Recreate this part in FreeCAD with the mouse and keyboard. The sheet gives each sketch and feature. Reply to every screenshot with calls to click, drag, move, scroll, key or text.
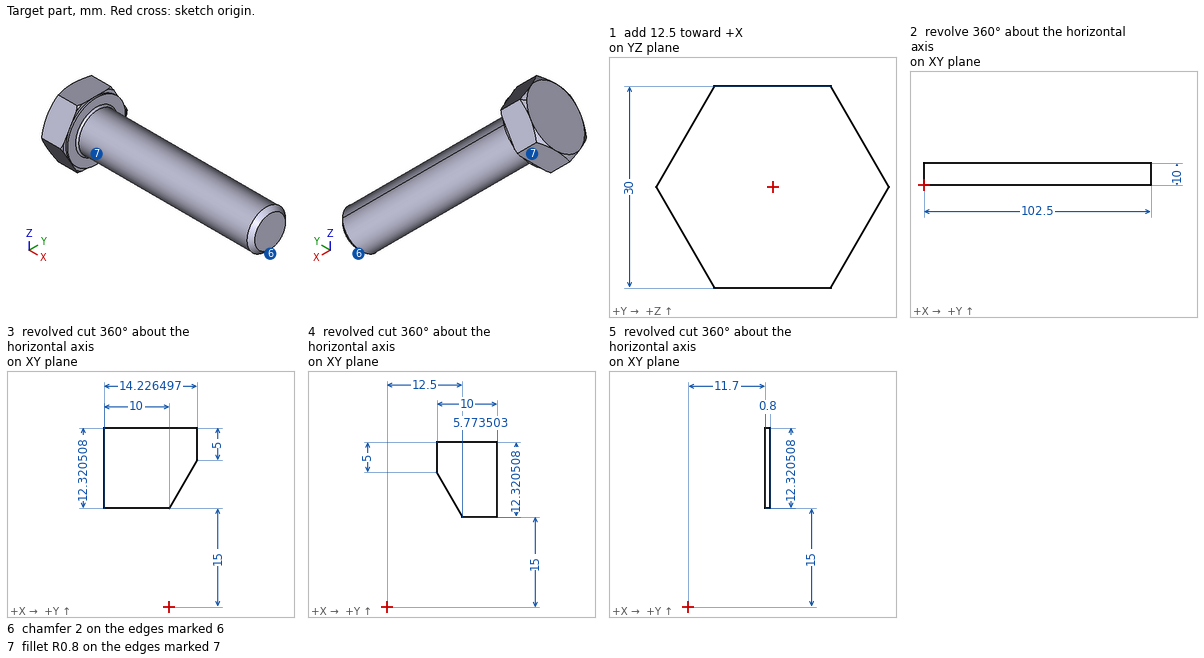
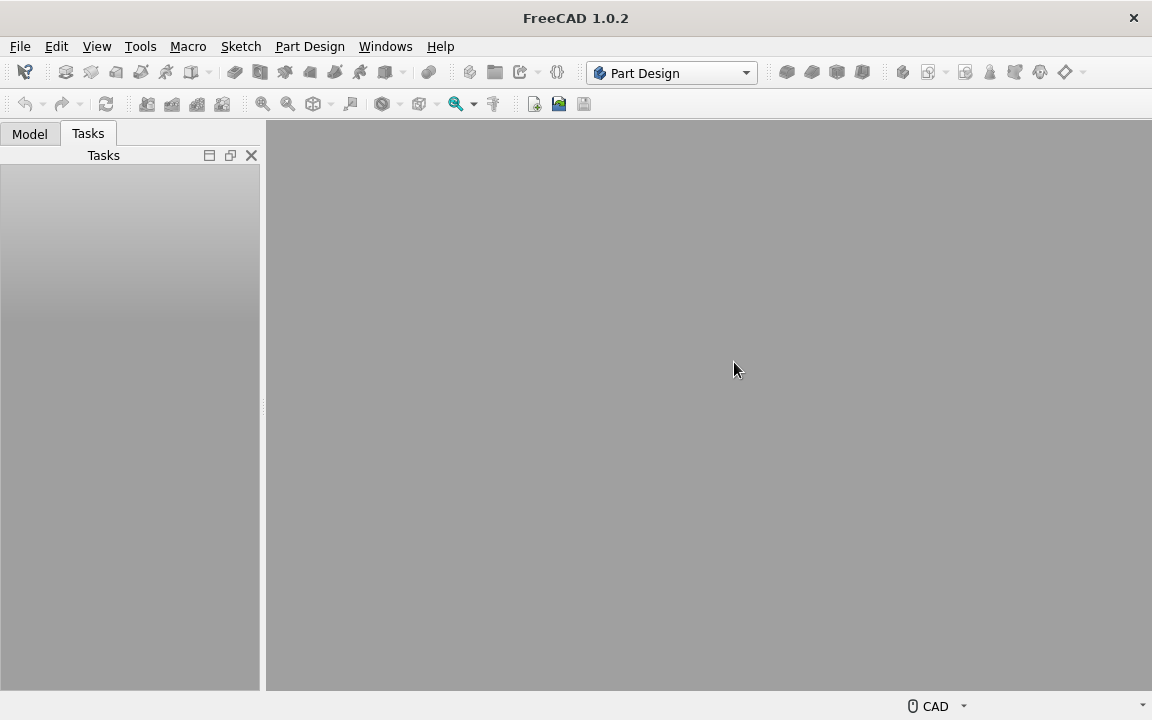
click(534, 104)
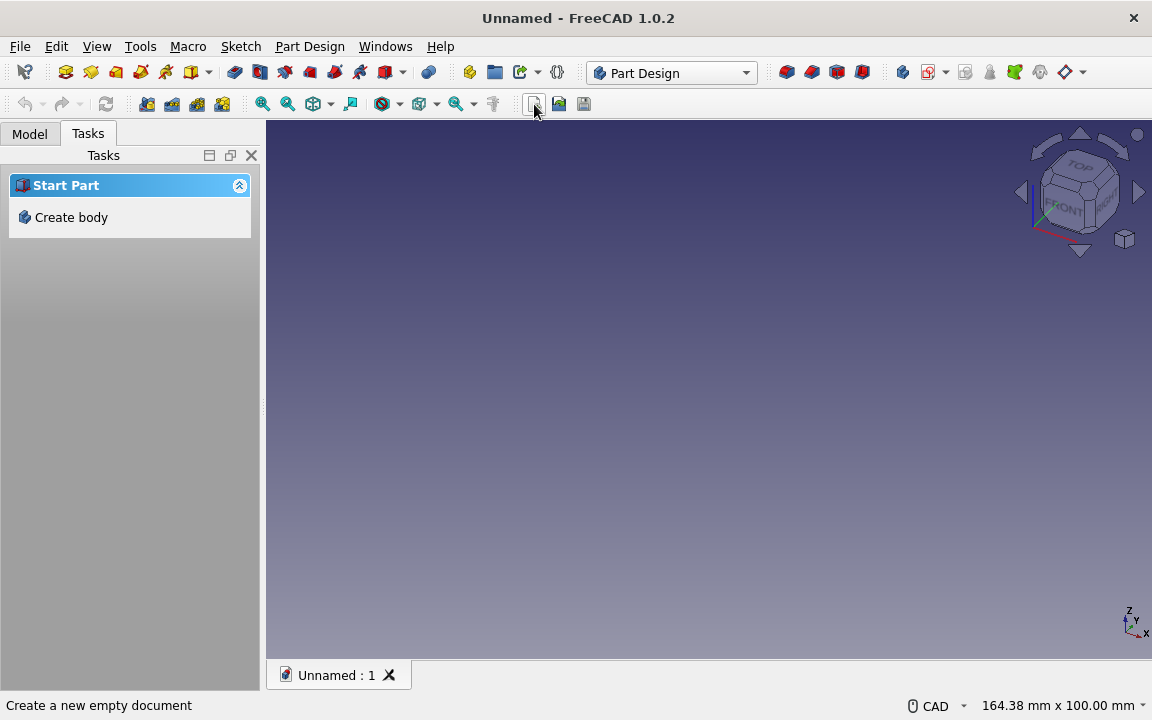
click(928, 72)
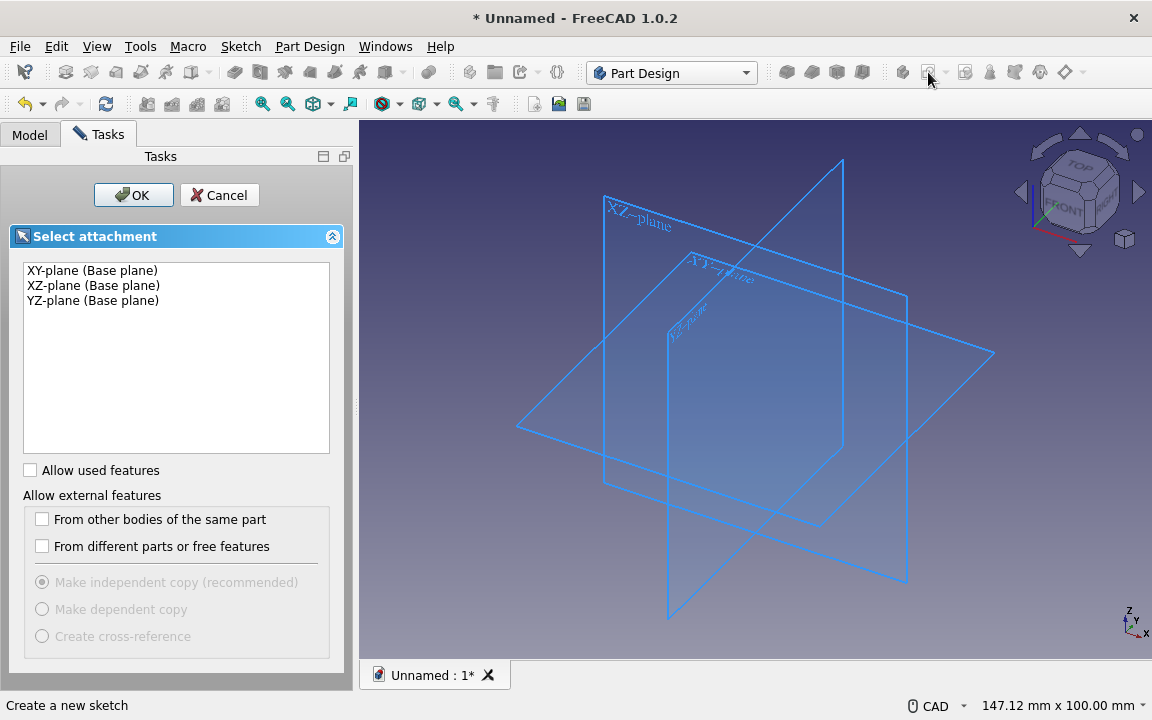
click(84, 300)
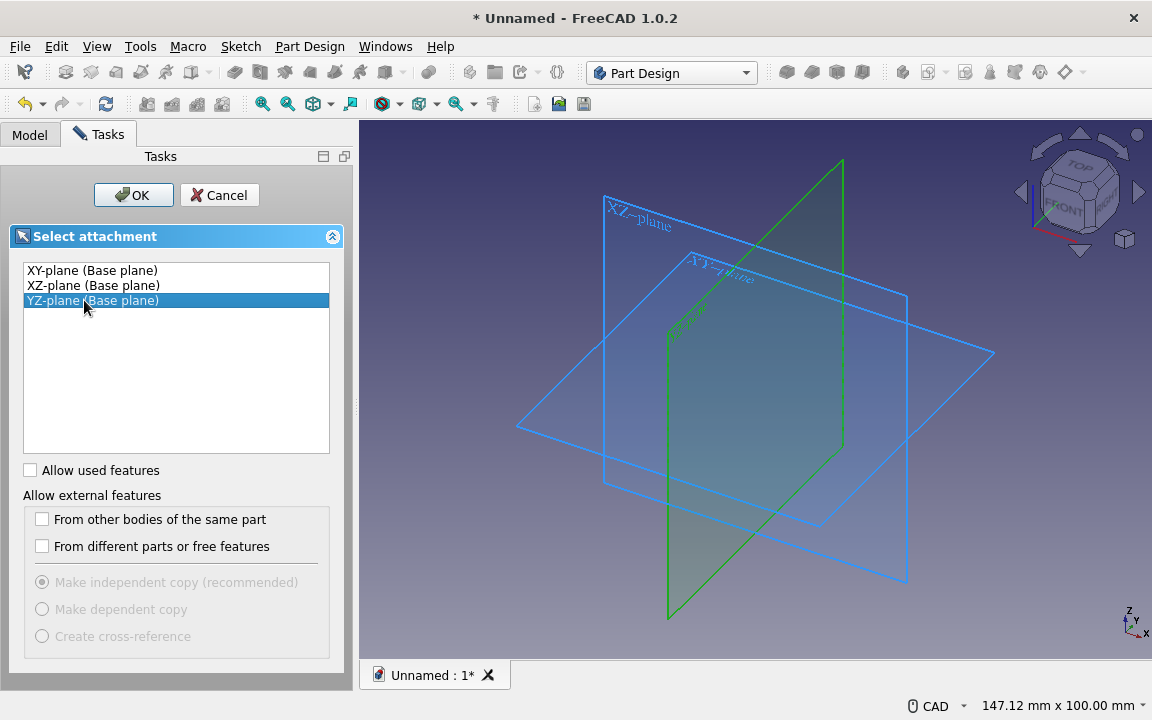
click(134, 195)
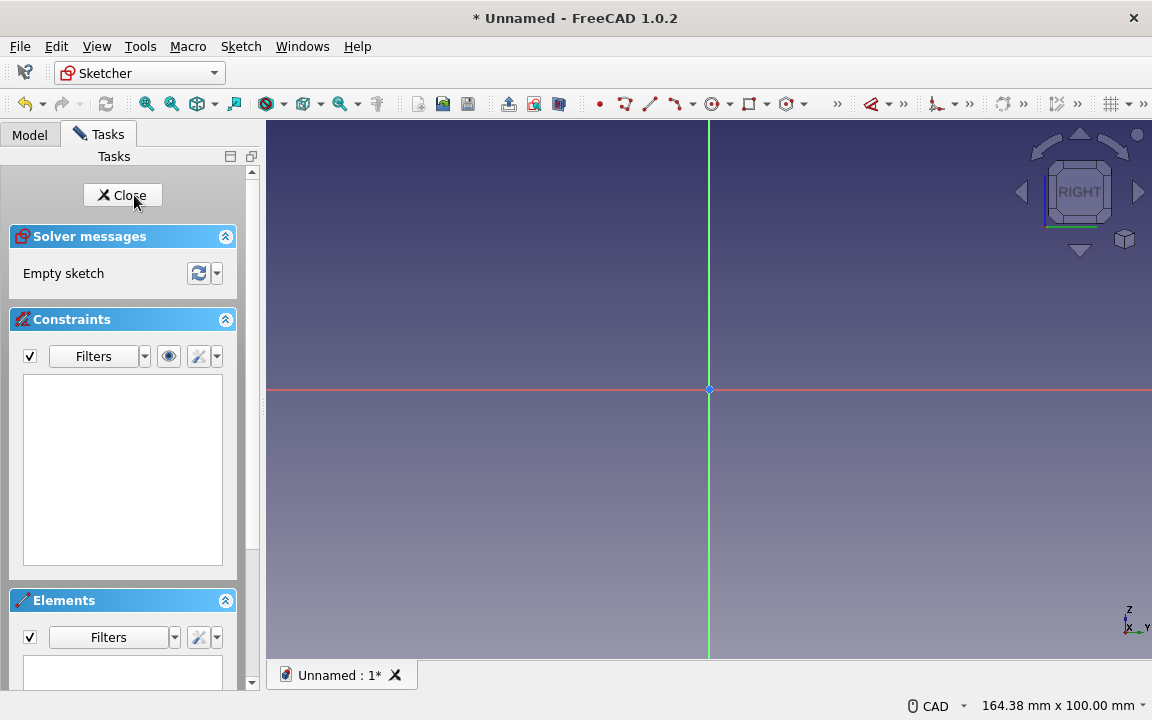
scroll(765, 390, up, 4)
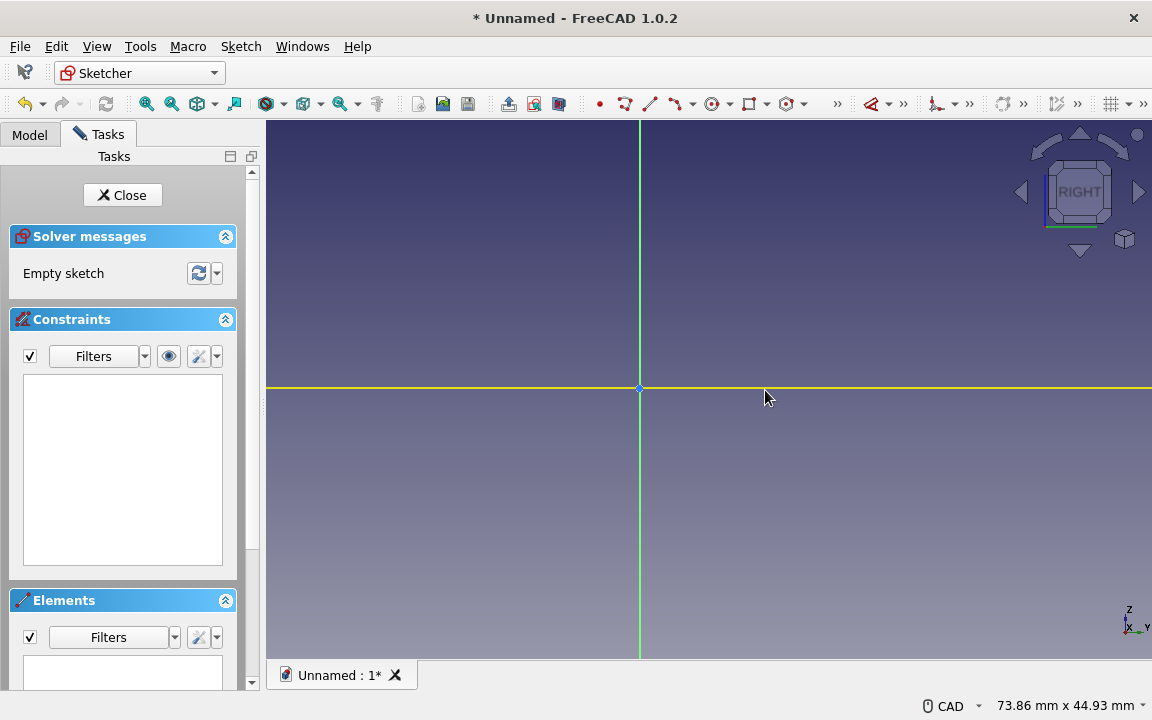
click(786, 104)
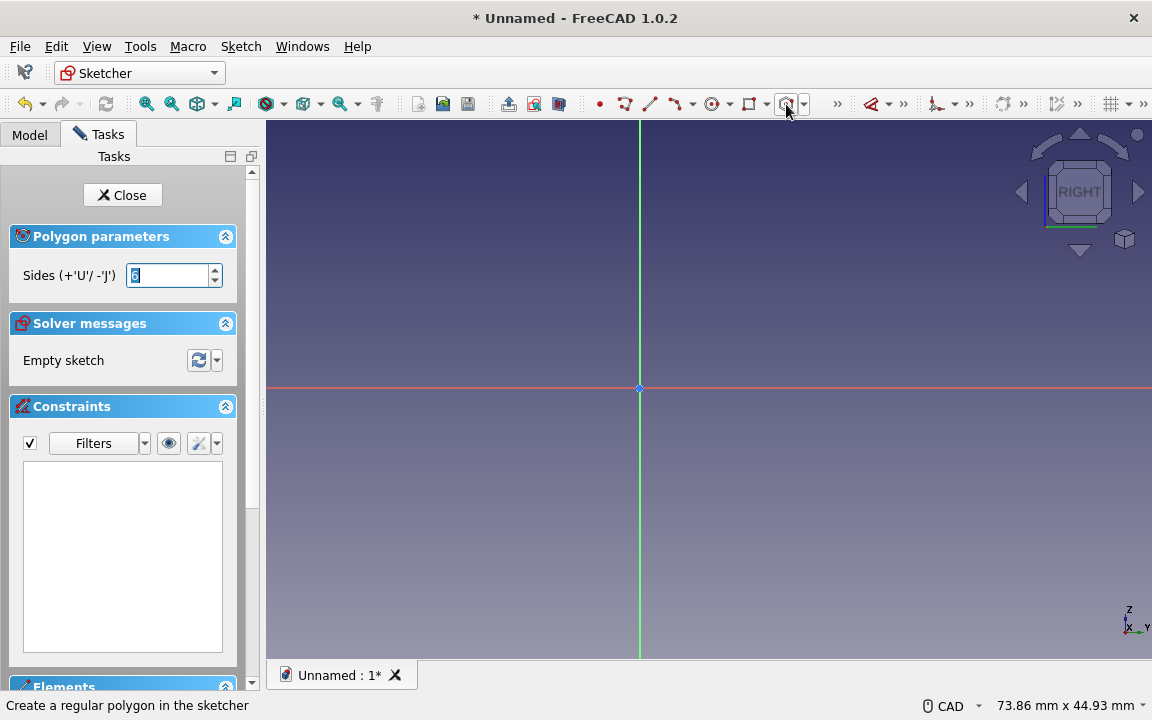
click(640, 388)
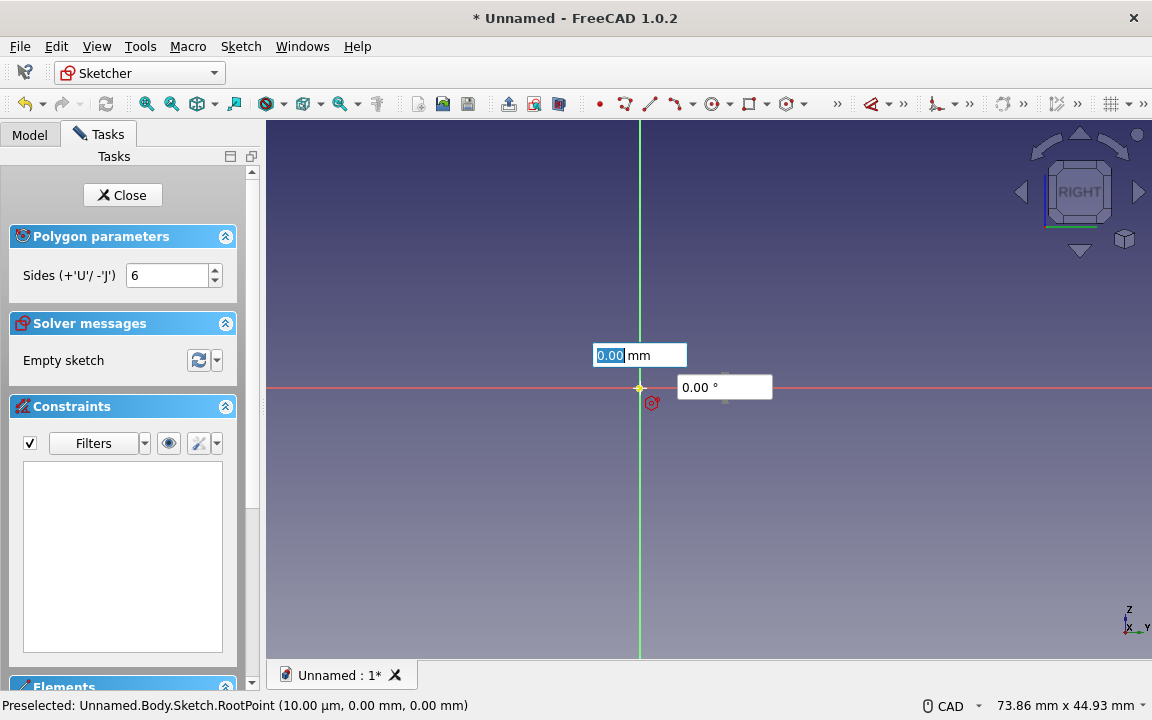
click(847, 388)
key(Escape)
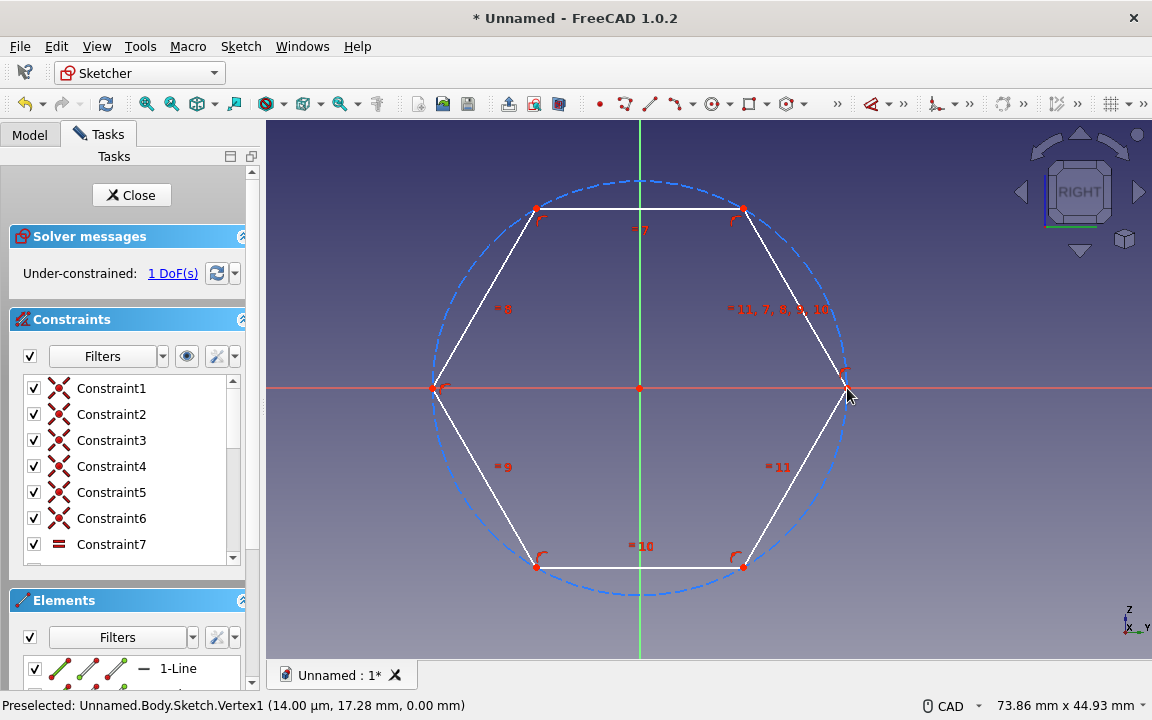
click(536, 568)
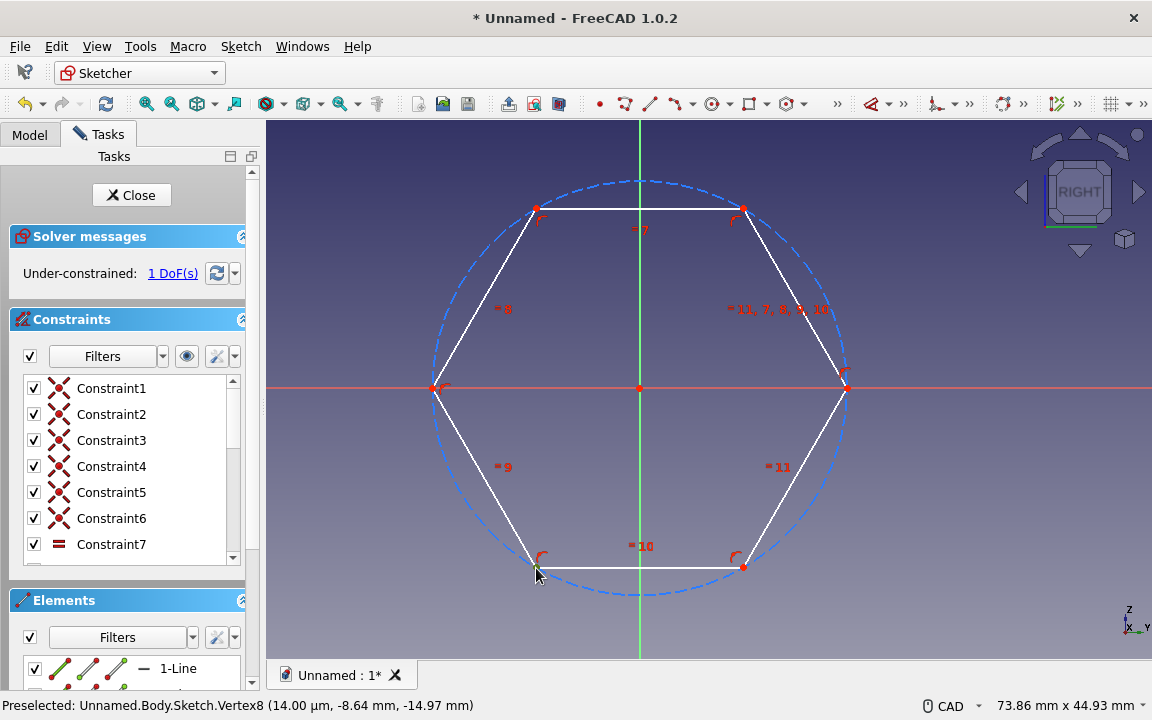
click(743, 209)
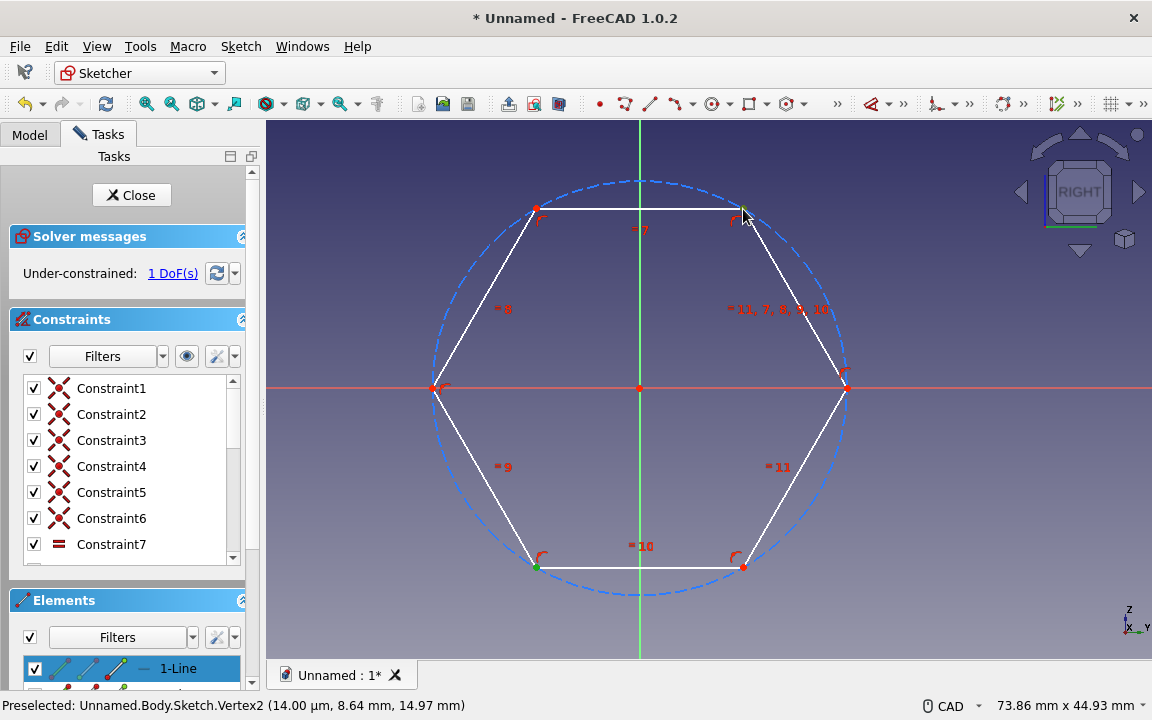
key(i)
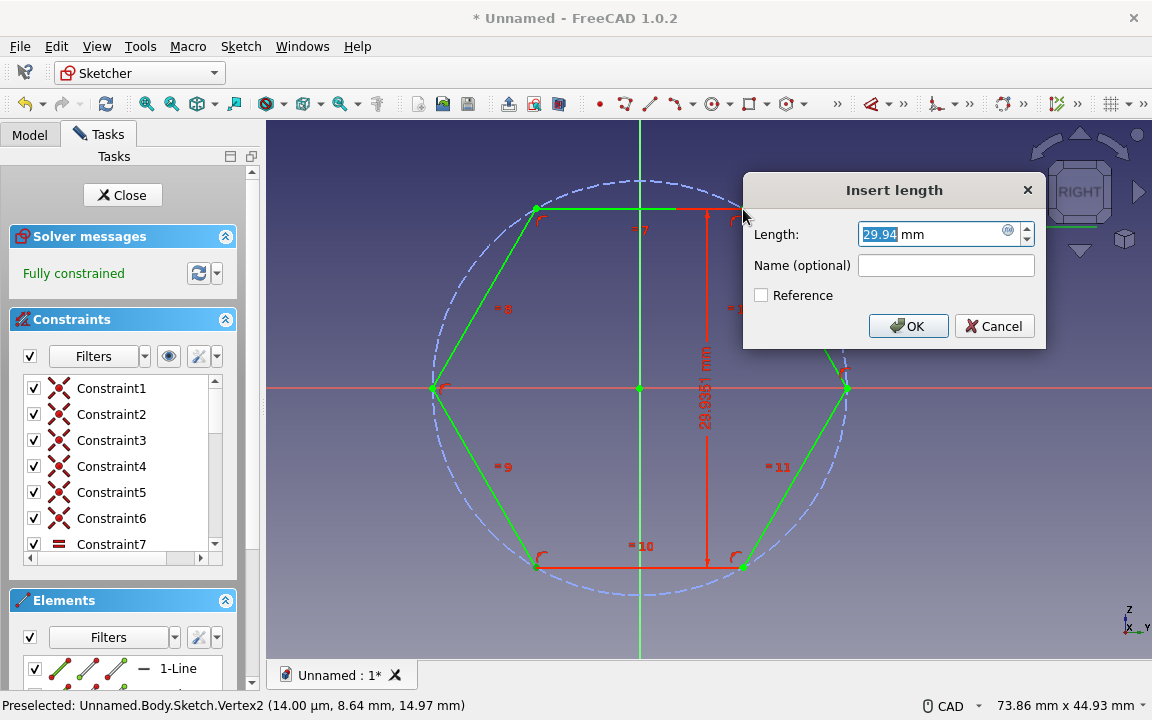
text(30)
key(Return)